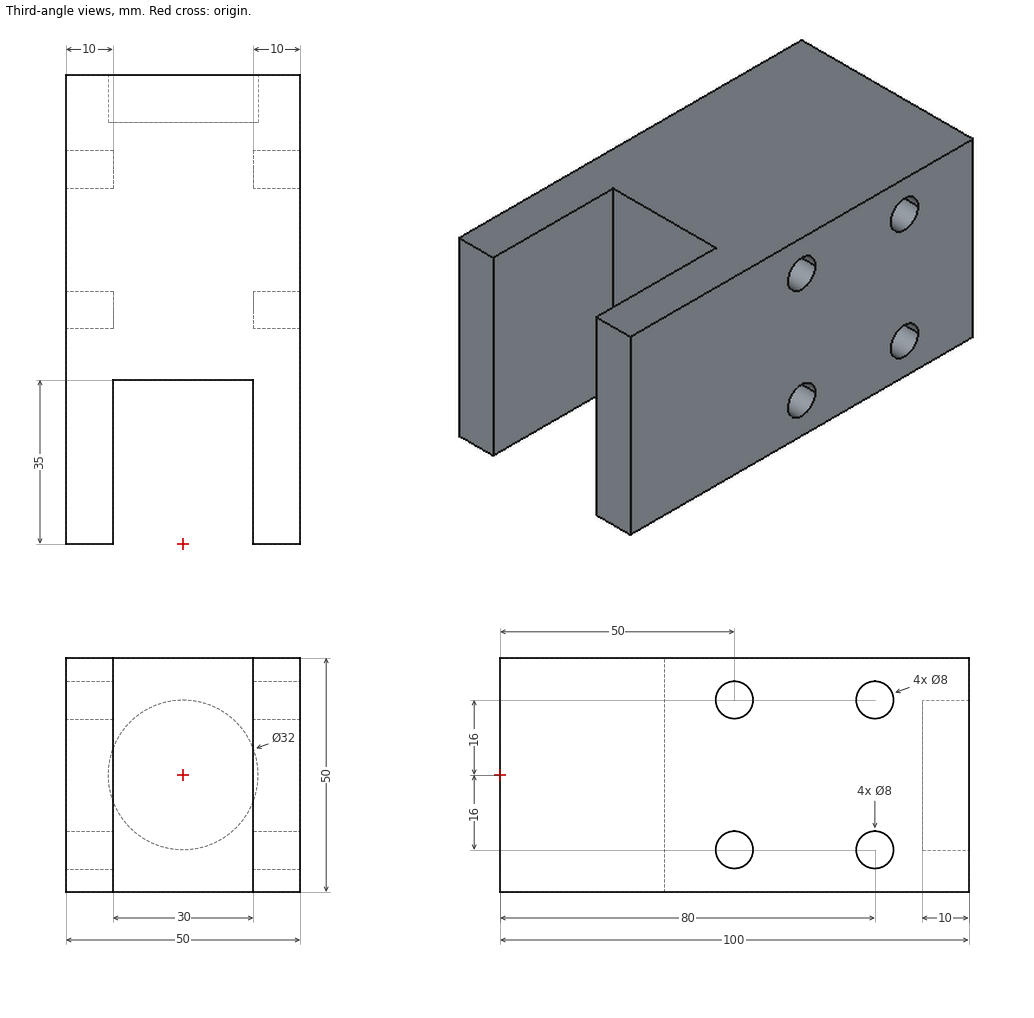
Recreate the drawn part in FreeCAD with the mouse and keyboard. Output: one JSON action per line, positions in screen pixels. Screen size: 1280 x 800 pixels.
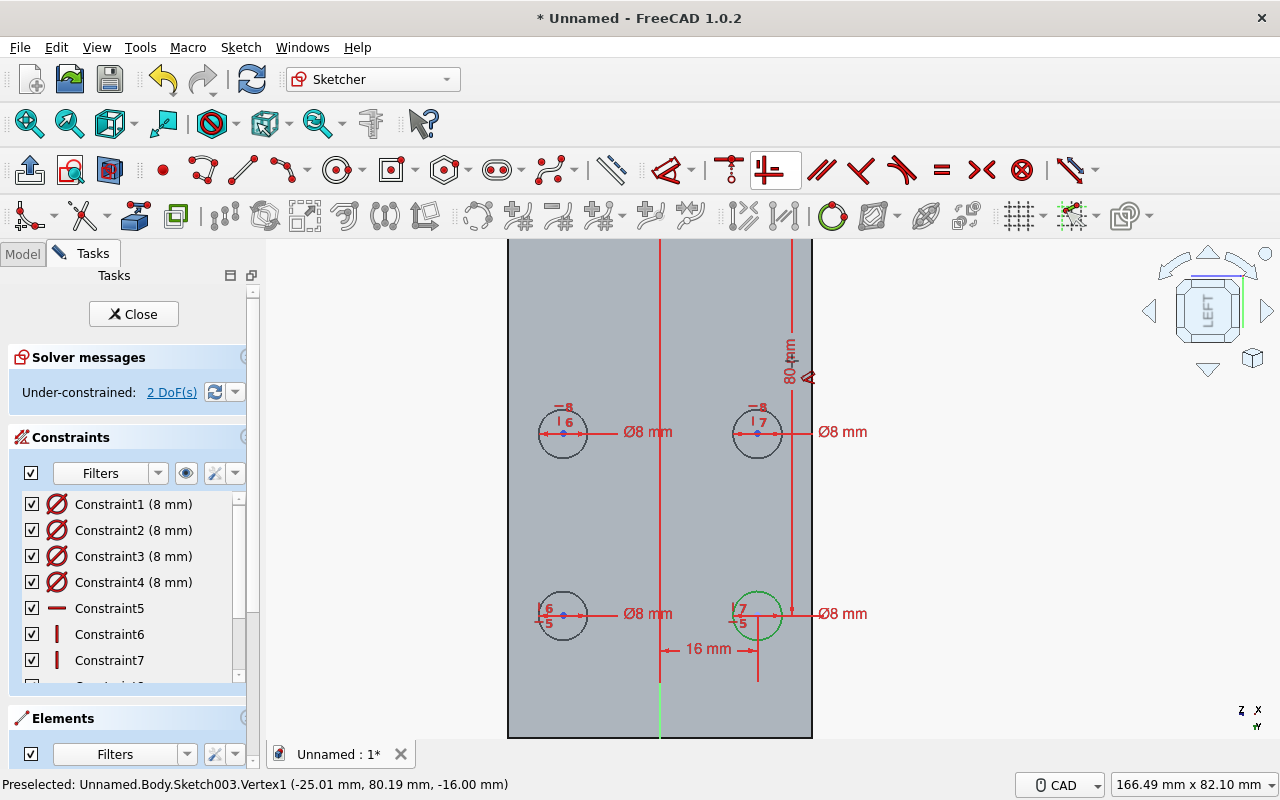
{"action": "left_click", "coordinate": [563, 616]}
{"action": "left_click", "coordinate": [612, 650]}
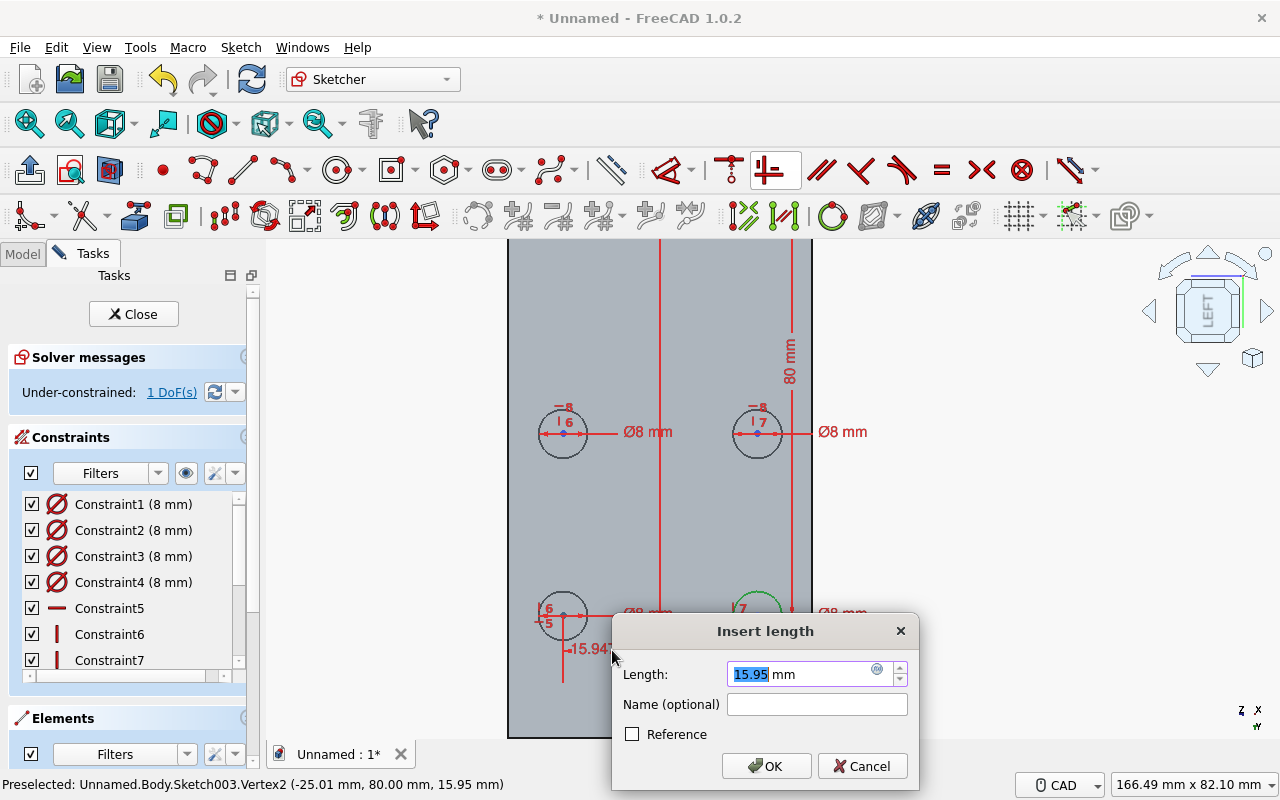
{"action": "type", "text": "16"}
{"action": "key", "text": "Return"}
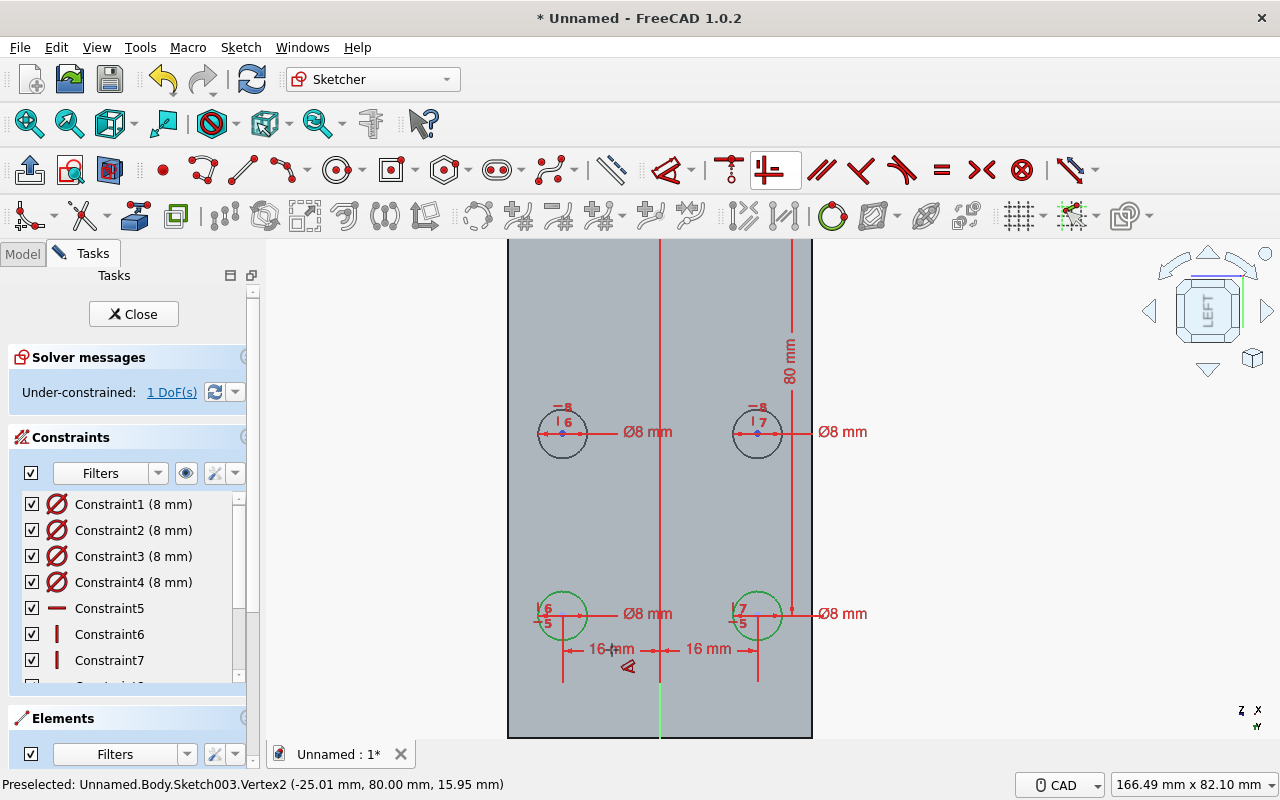
{"action": "left_click", "coordinate": [563, 434]}
{"action": "left_click", "coordinate": [529, 350]}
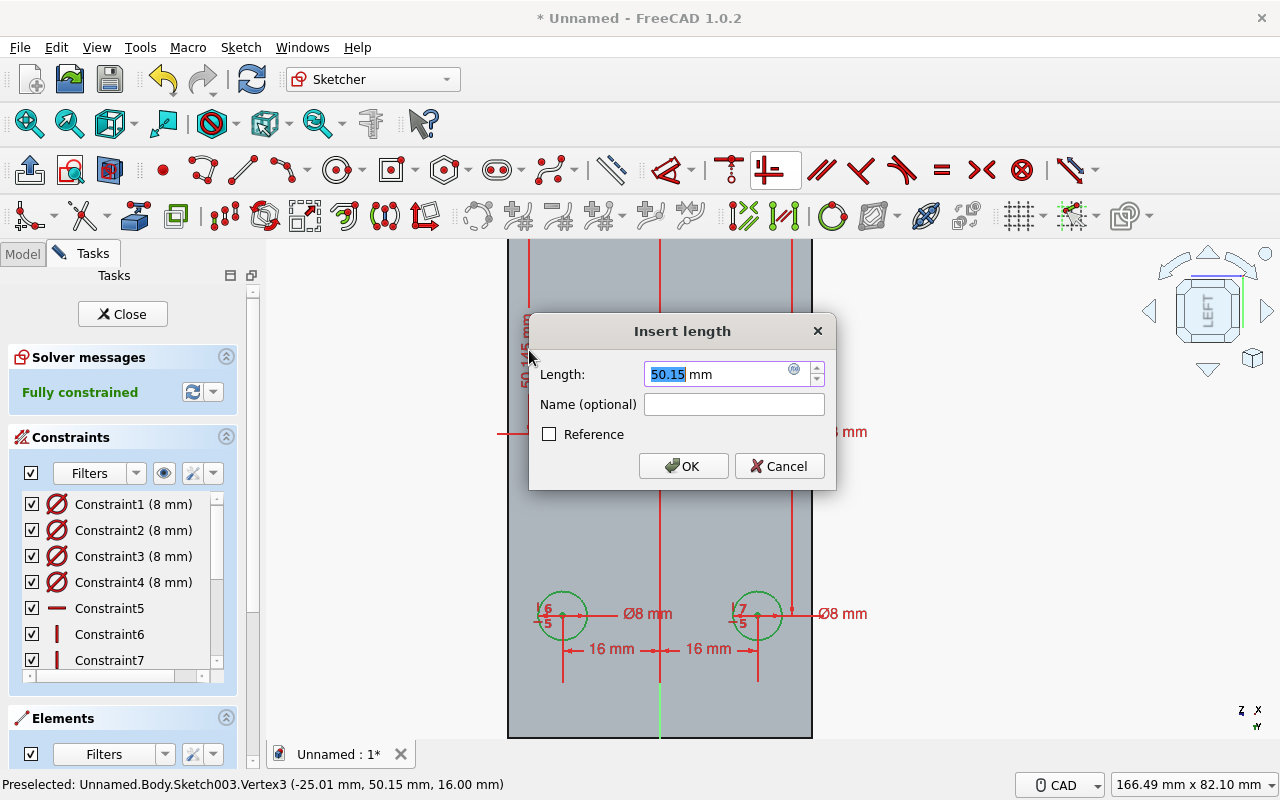
{"action": "type", "text": "50"}
{"action": "key", "text": "Return"}
{"action": "key", "text": "Escape"}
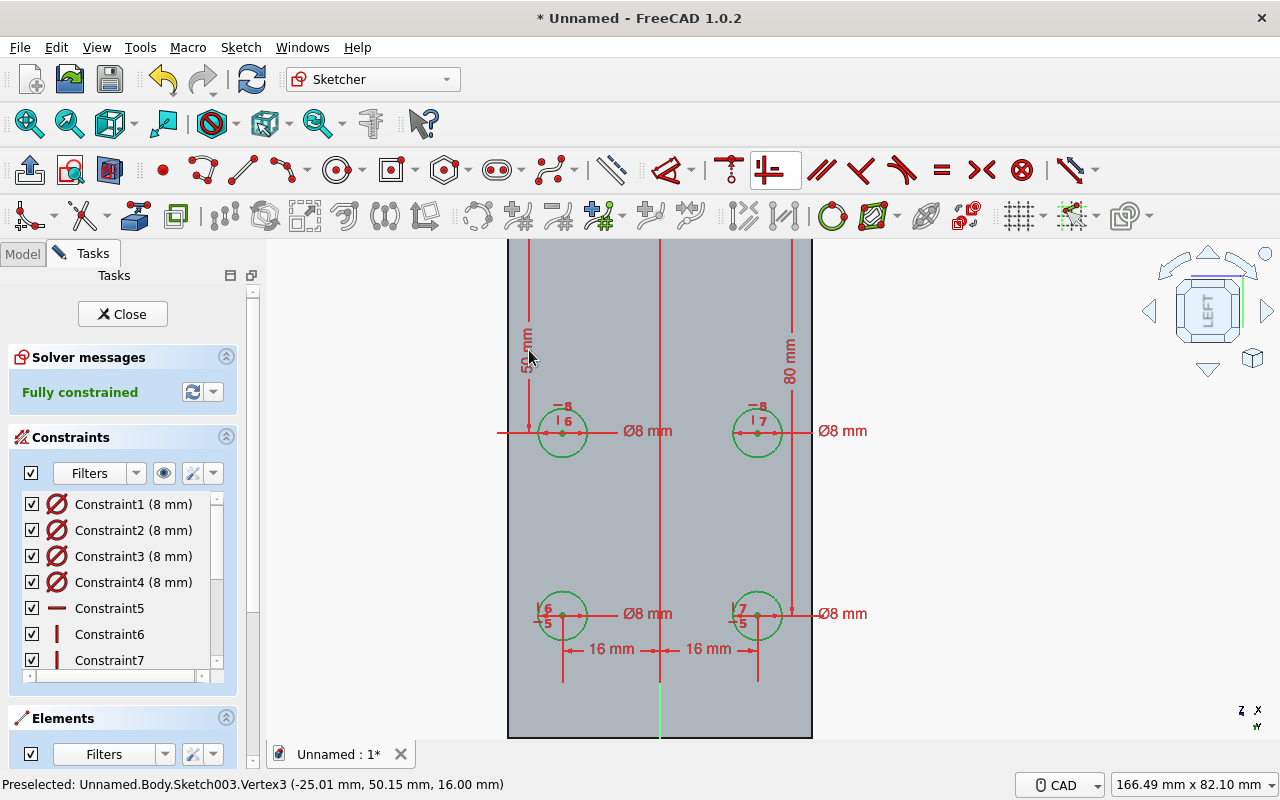
{"action": "left_click", "coordinate": [123, 314]}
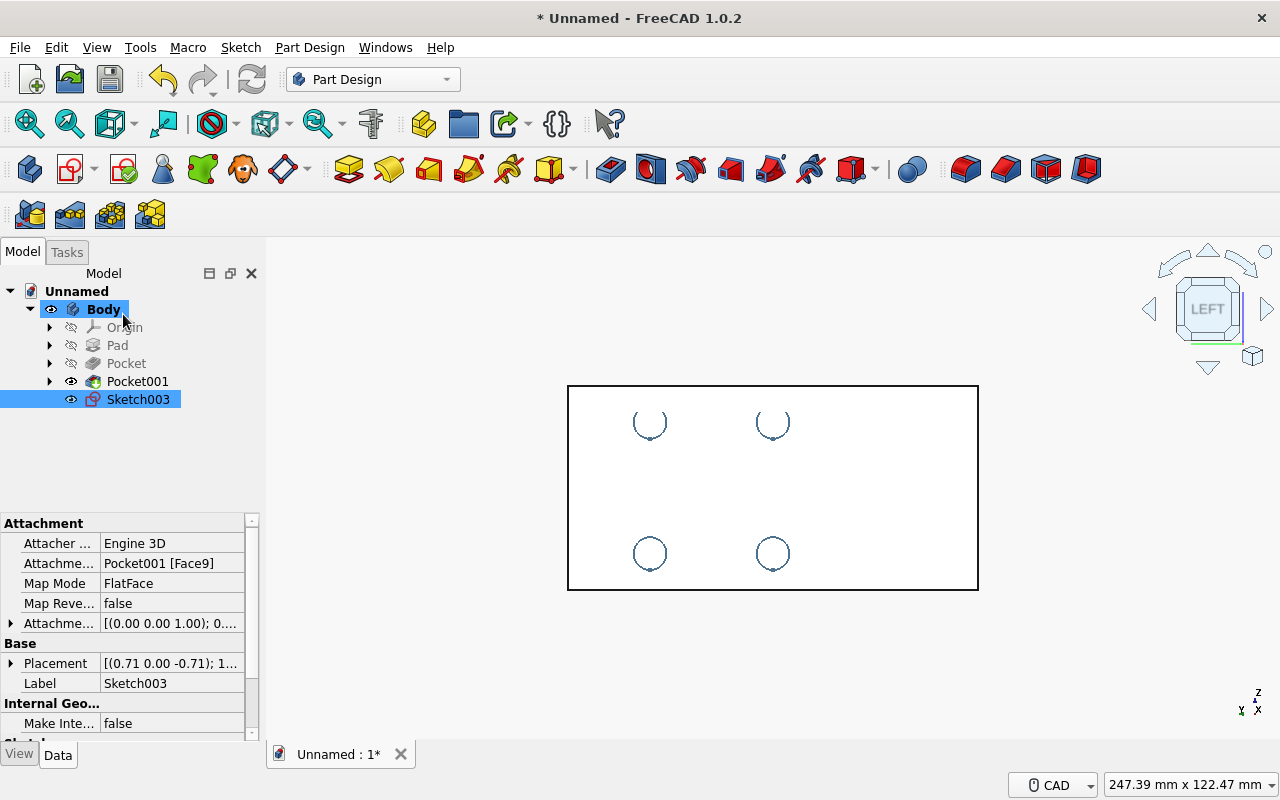
{"action": "left_click", "coordinate": [612, 170]}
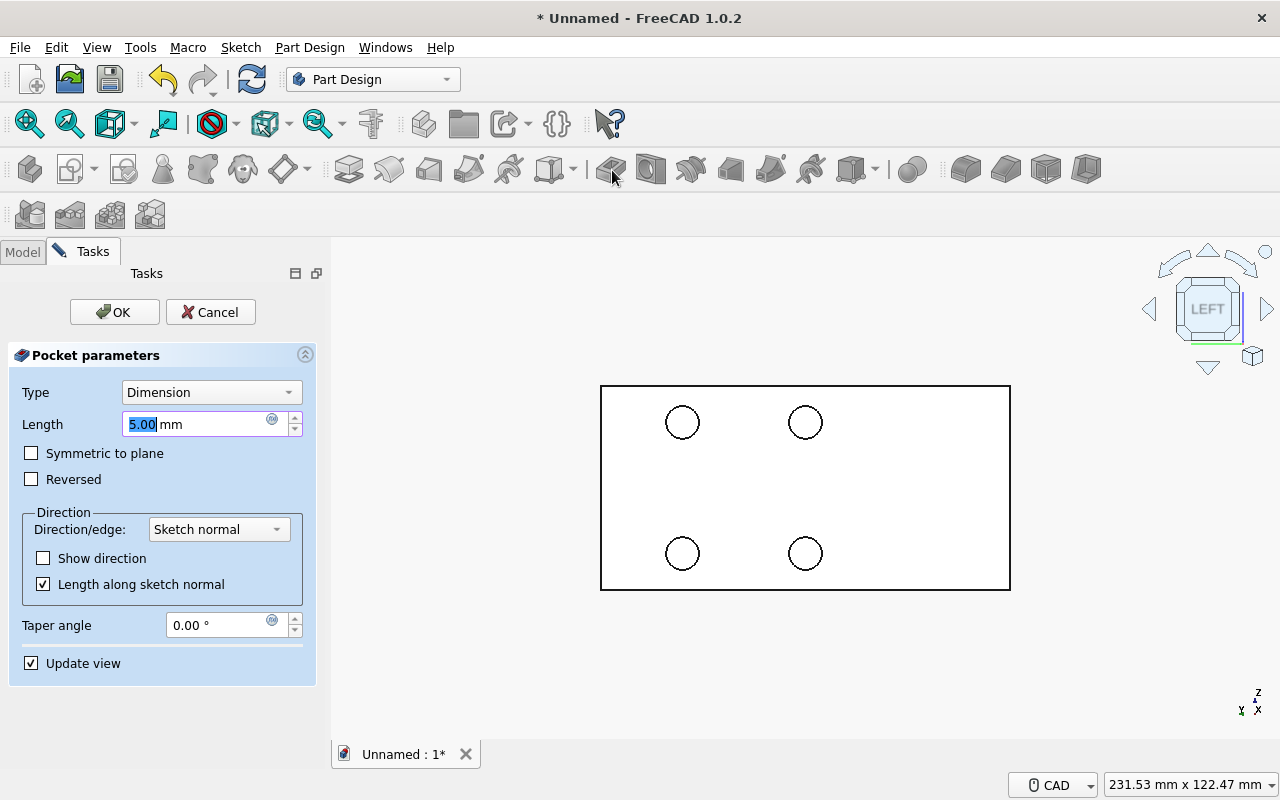
{"action": "type", "text": "10"}
{"action": "key", "text": "Tab"}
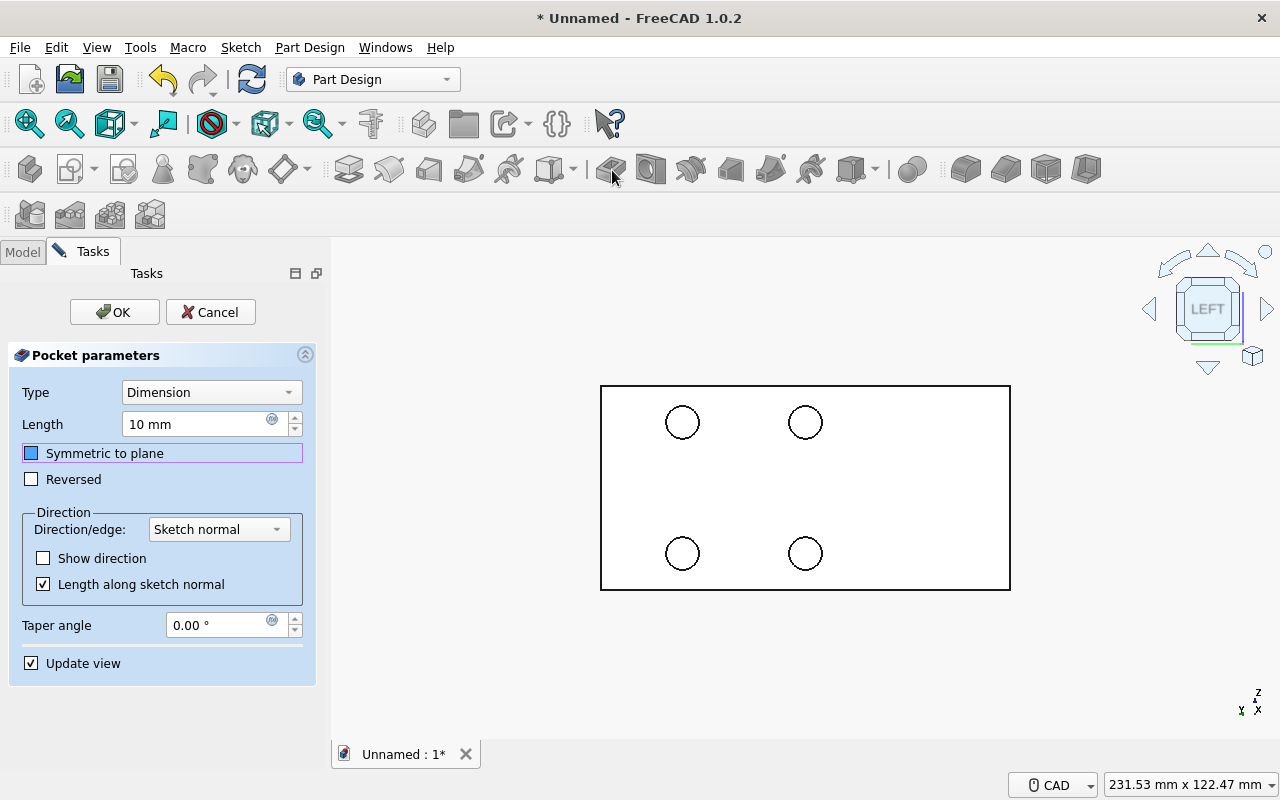
{"action": "left_click", "coordinate": [115, 312]}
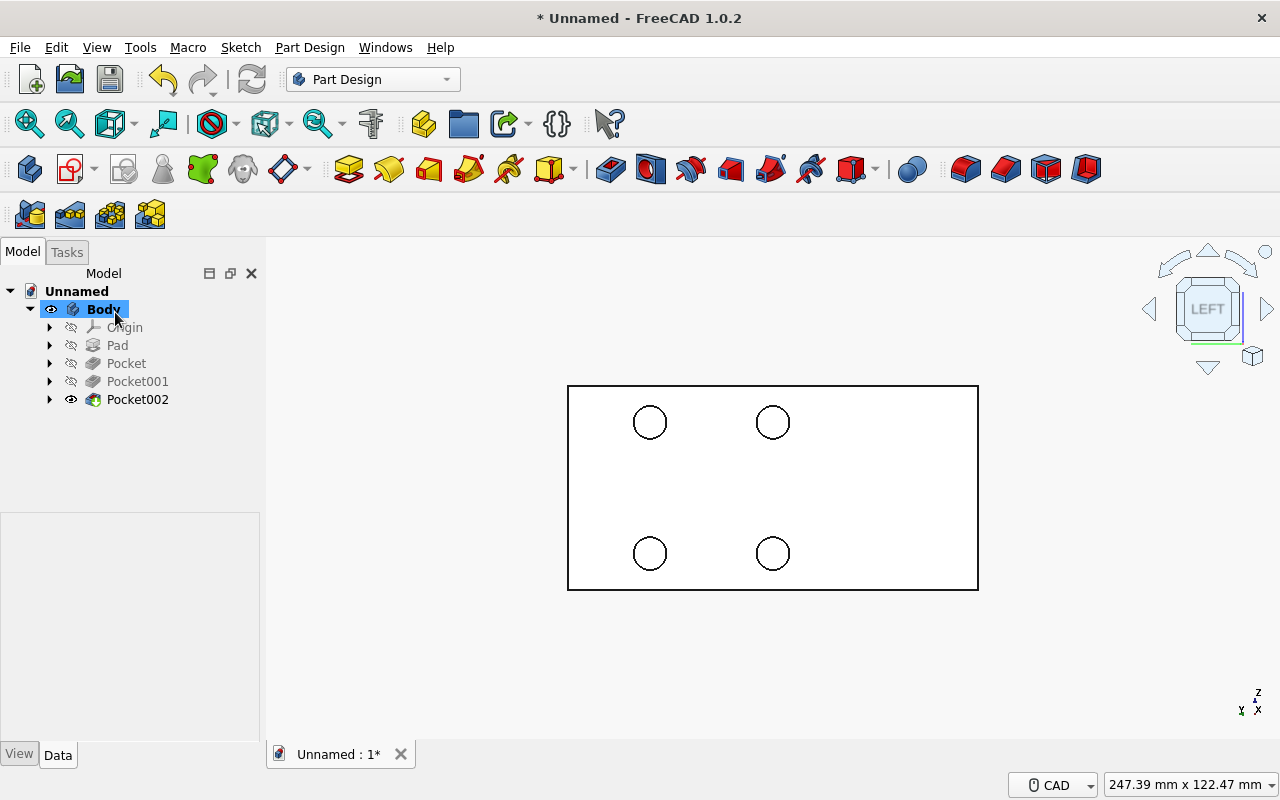
{"action": "left_click", "coordinate": [30, 124]}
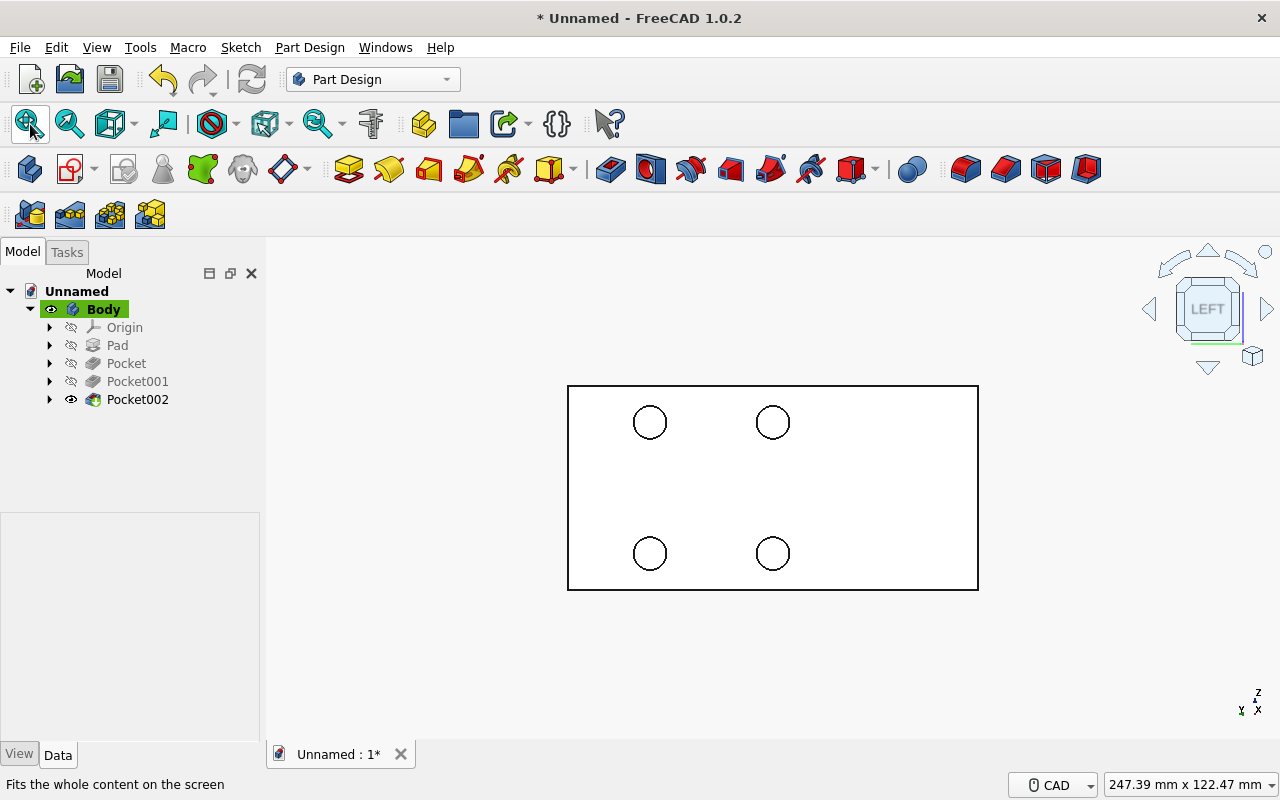
{"action": "left_click", "coordinate": [50, 327]}